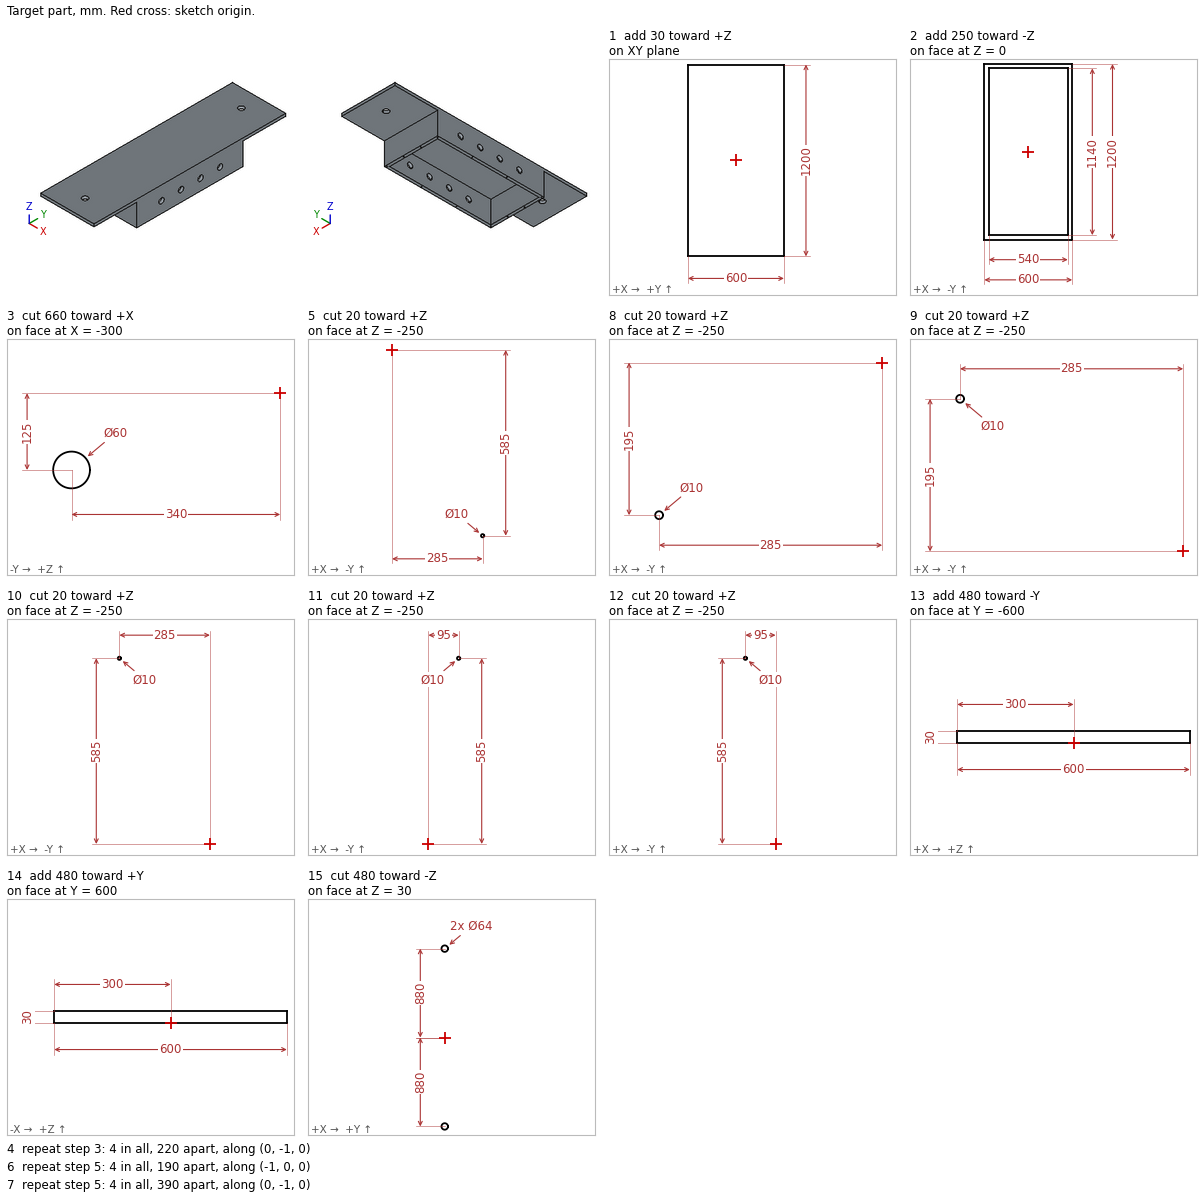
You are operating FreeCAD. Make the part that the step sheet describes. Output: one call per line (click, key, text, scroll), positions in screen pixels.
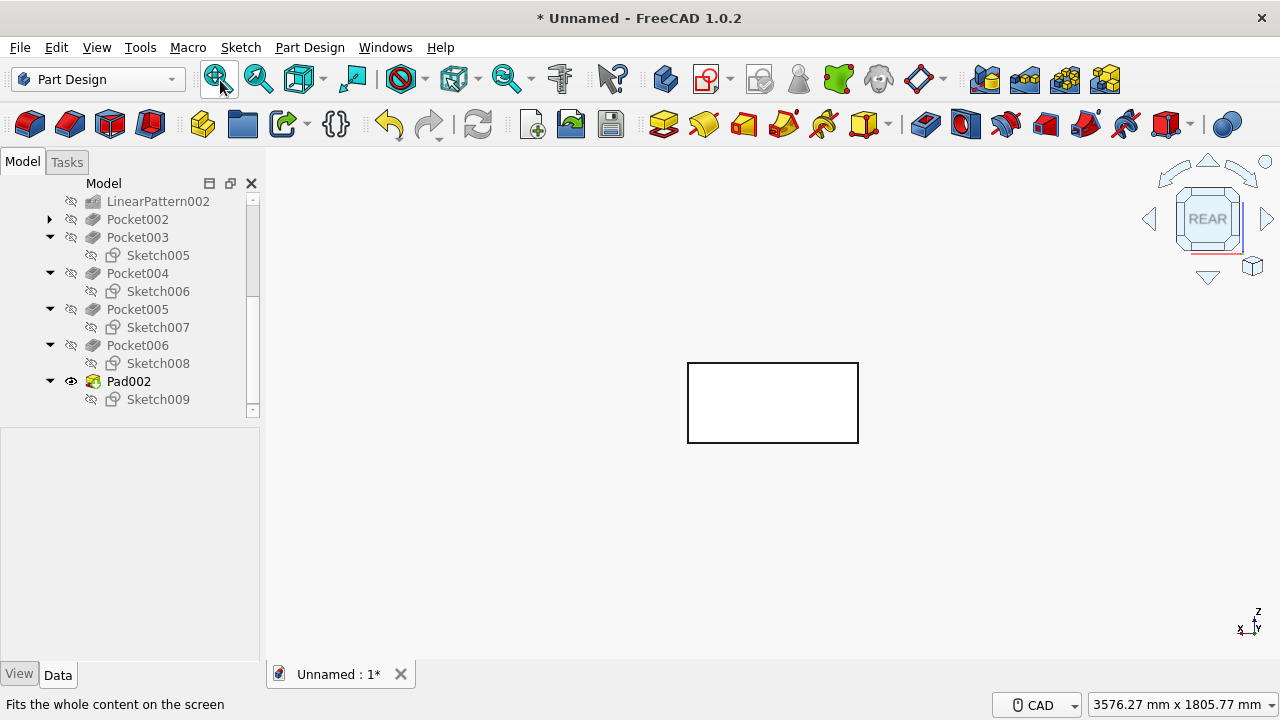
click(749, 402)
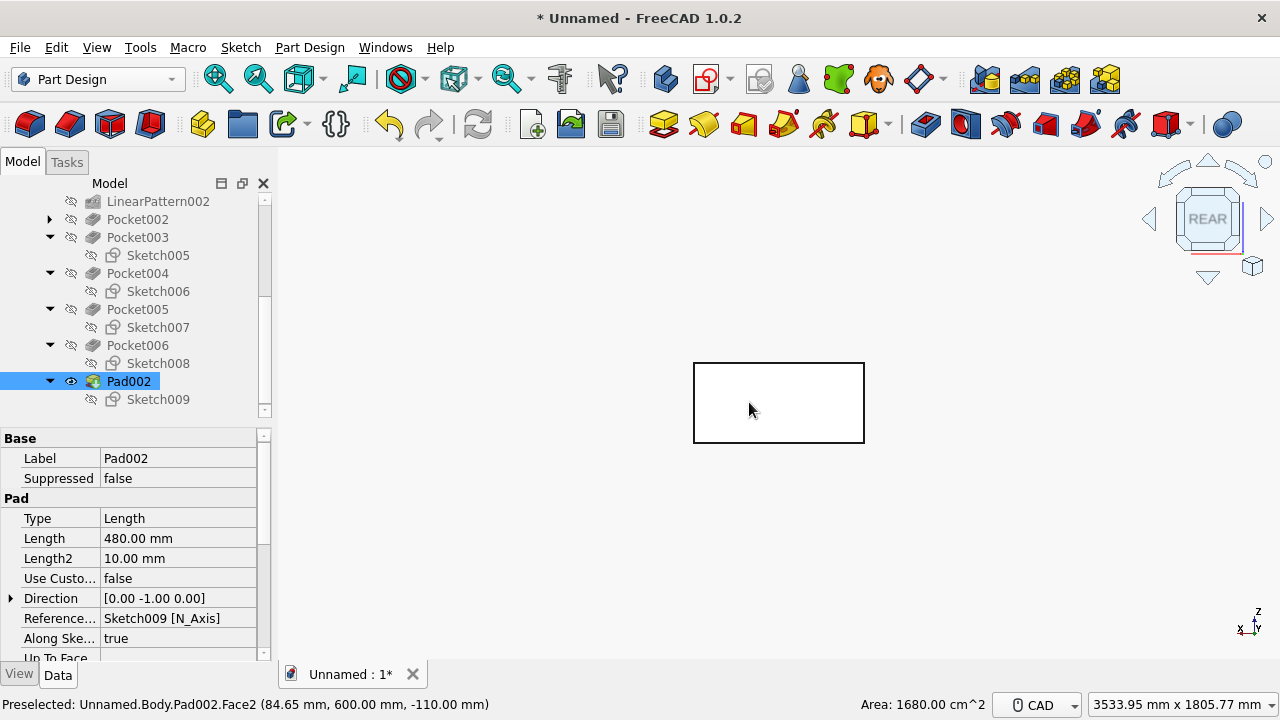
click(706, 80)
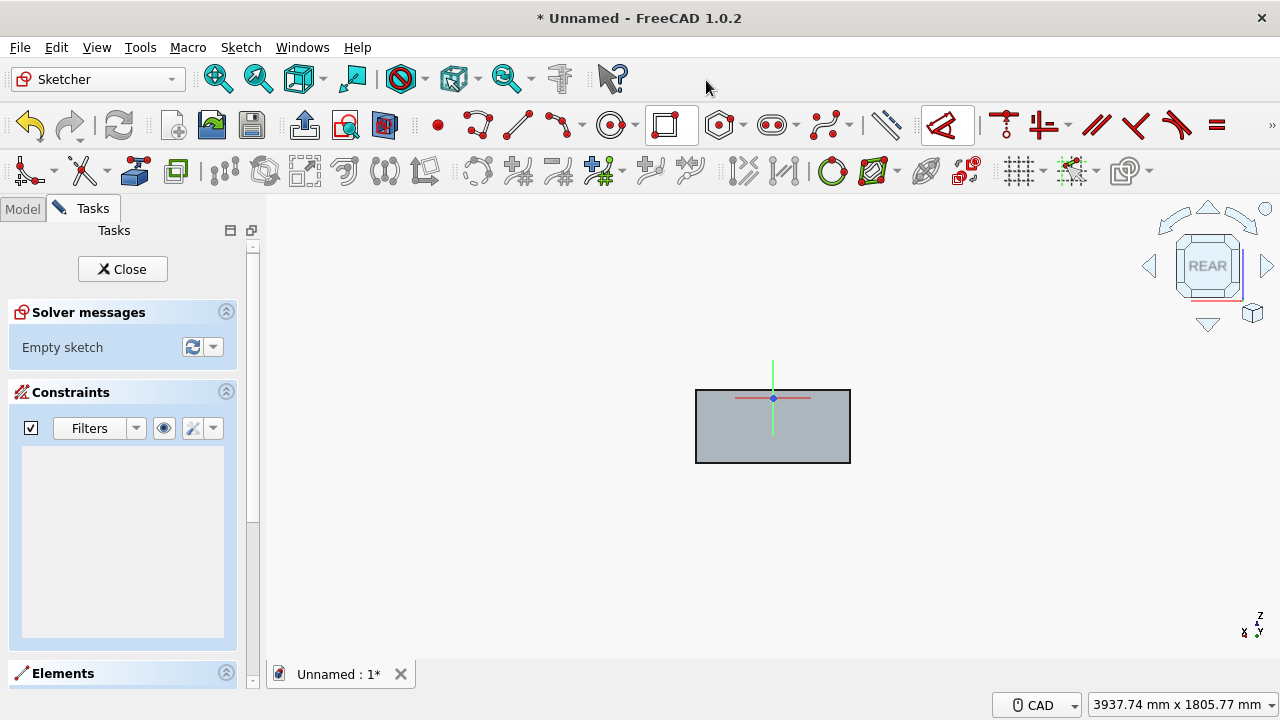
scroll(795, 384, up, 7)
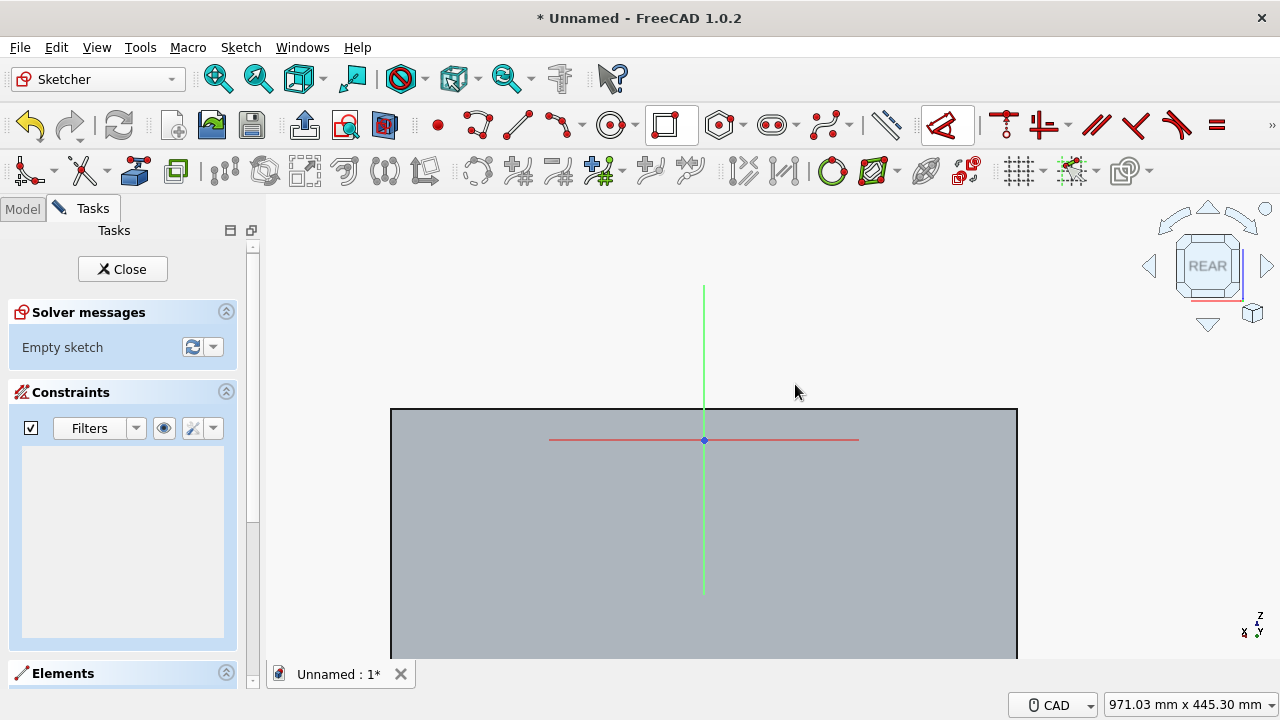
click(666, 126)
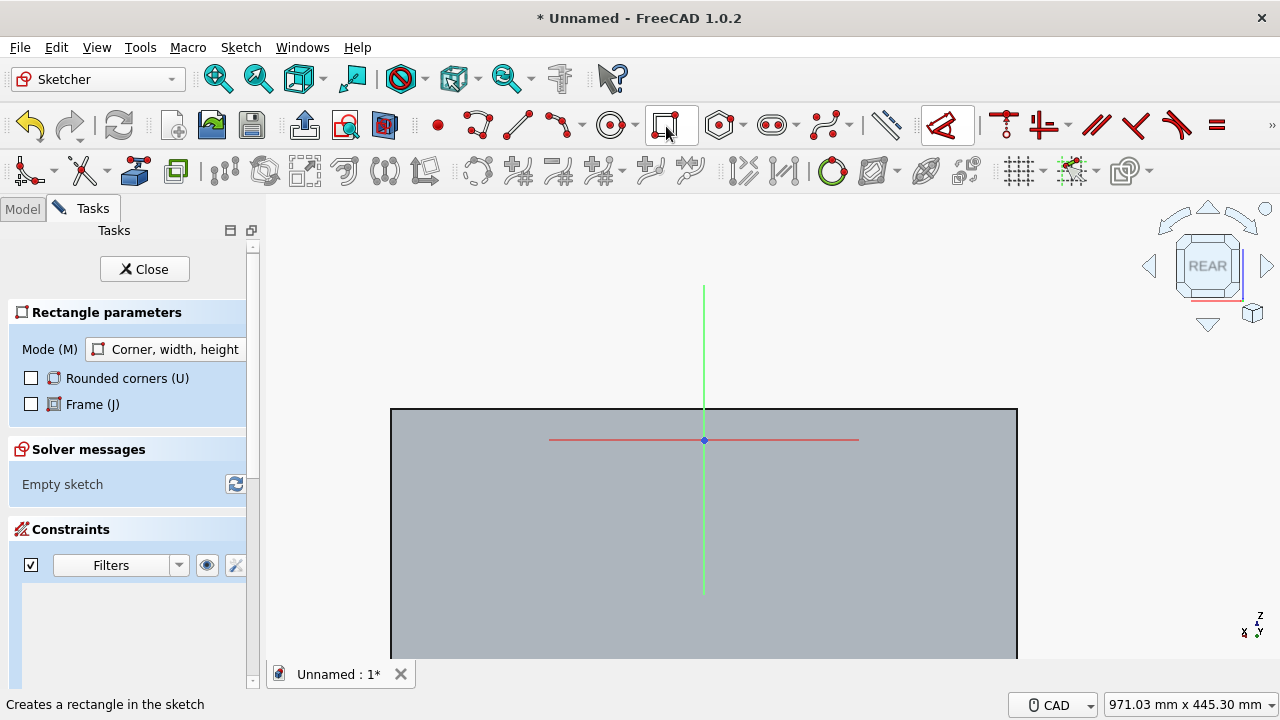
click(391, 409)
click(1017, 440)
key(Escape)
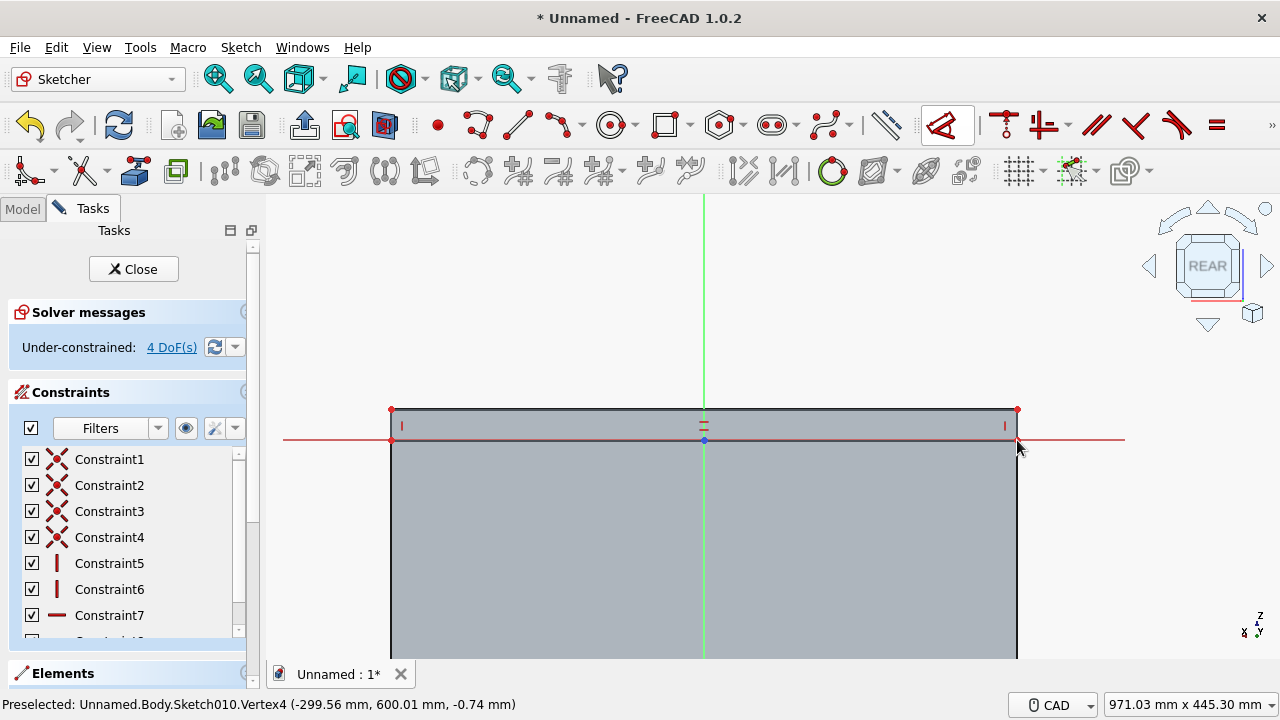
click(391, 441)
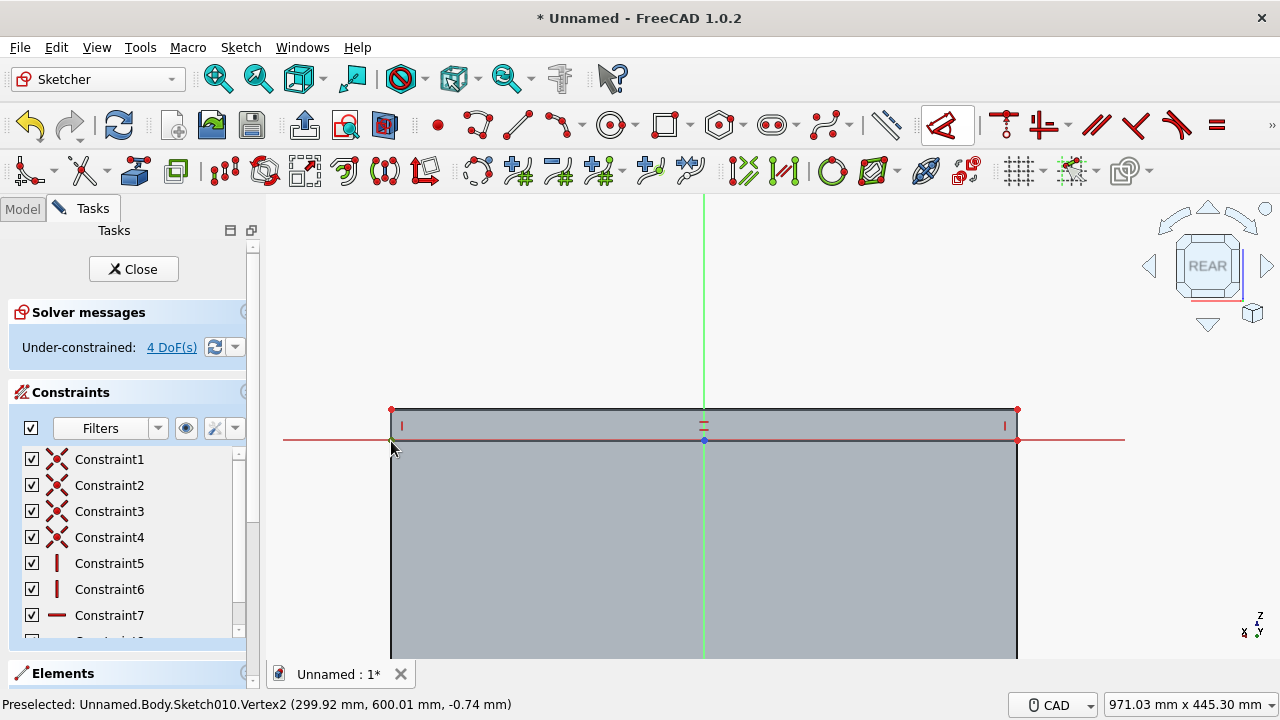
click(353, 440)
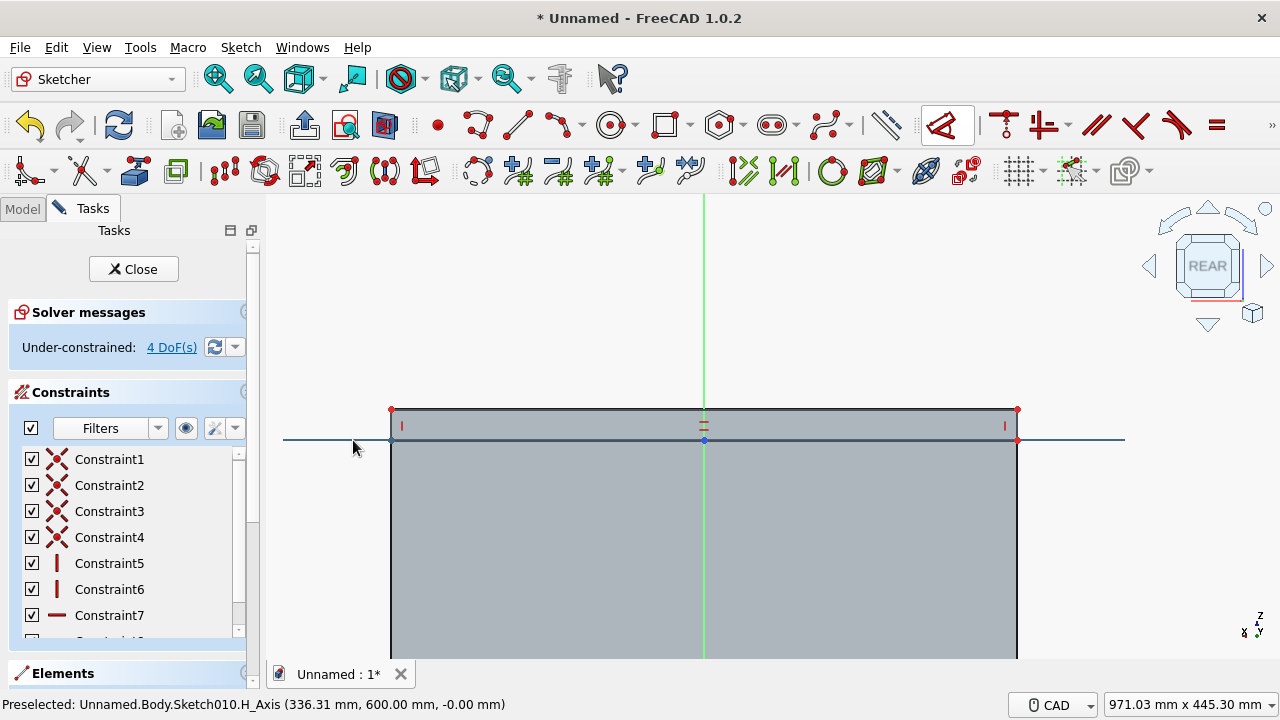
click(1004, 126)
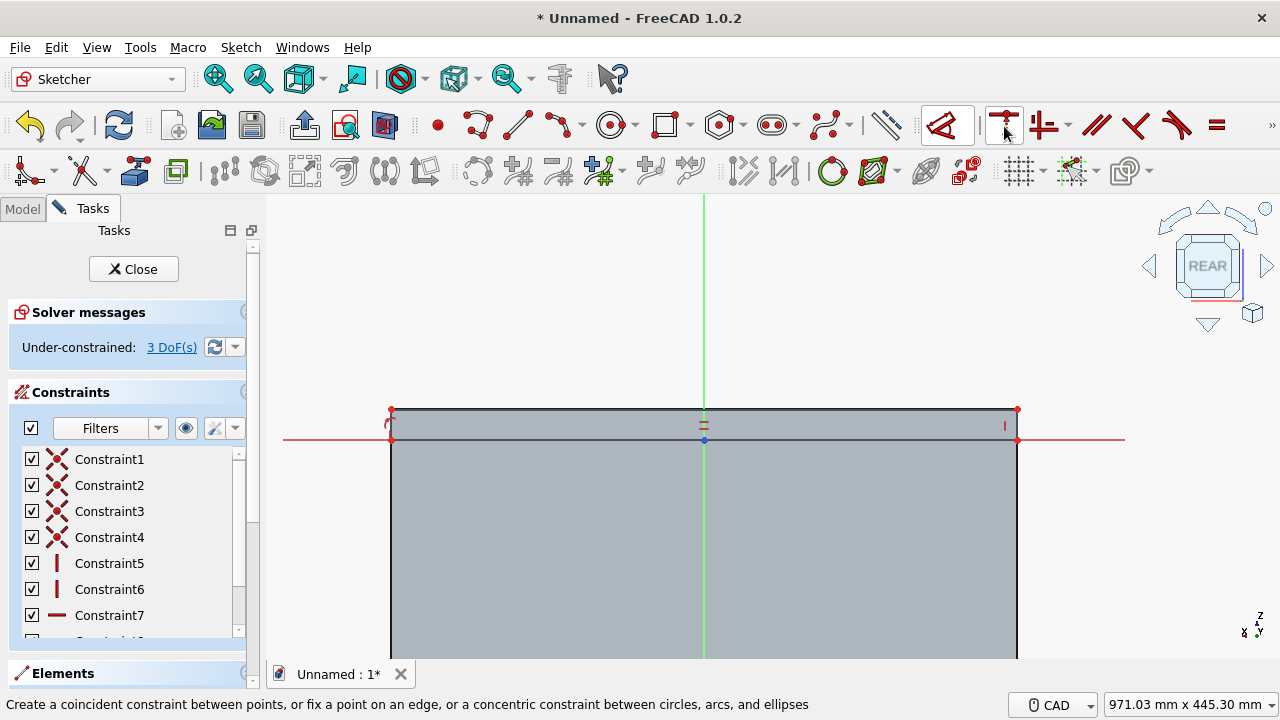
scroll(391, 419, up, 3)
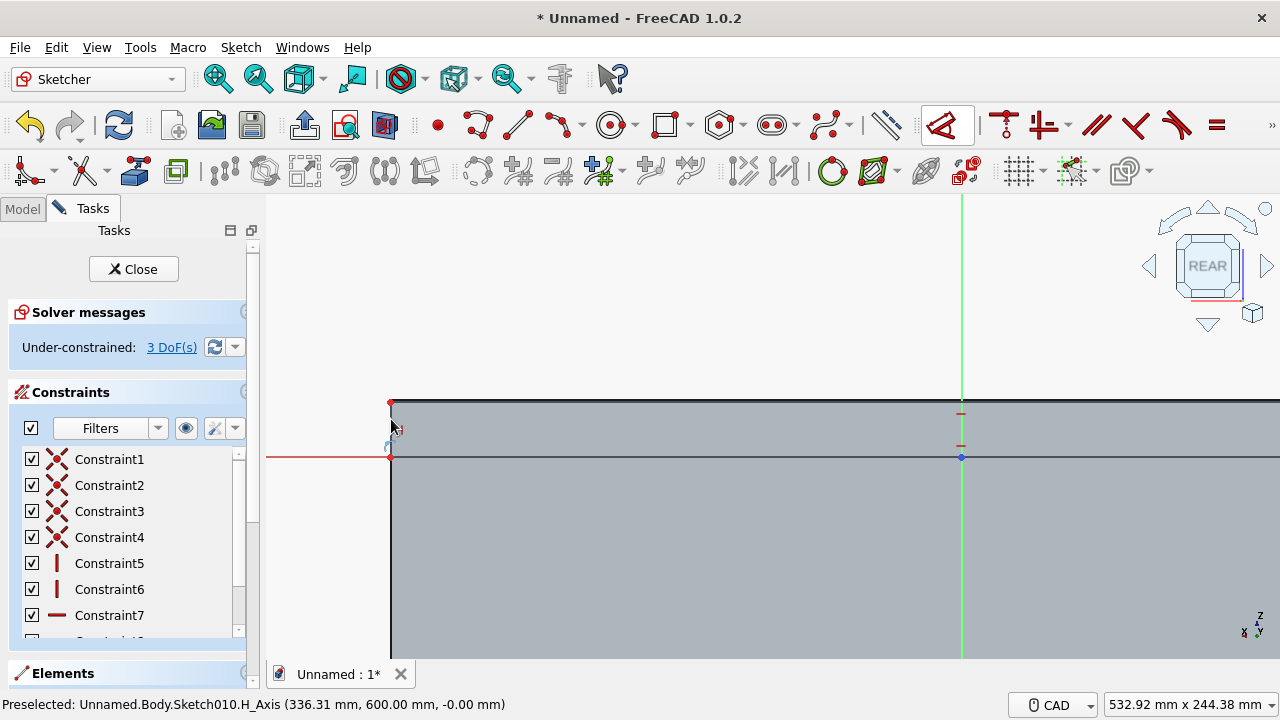
click(391, 419)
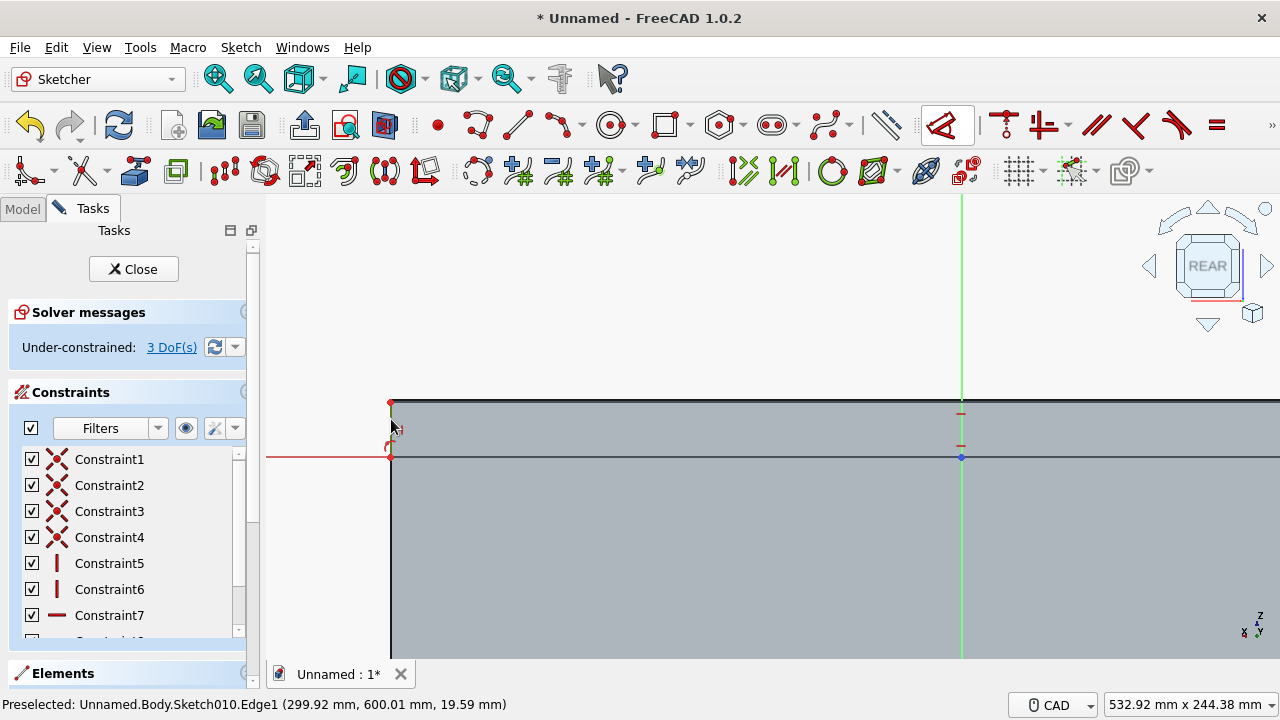
key(i)